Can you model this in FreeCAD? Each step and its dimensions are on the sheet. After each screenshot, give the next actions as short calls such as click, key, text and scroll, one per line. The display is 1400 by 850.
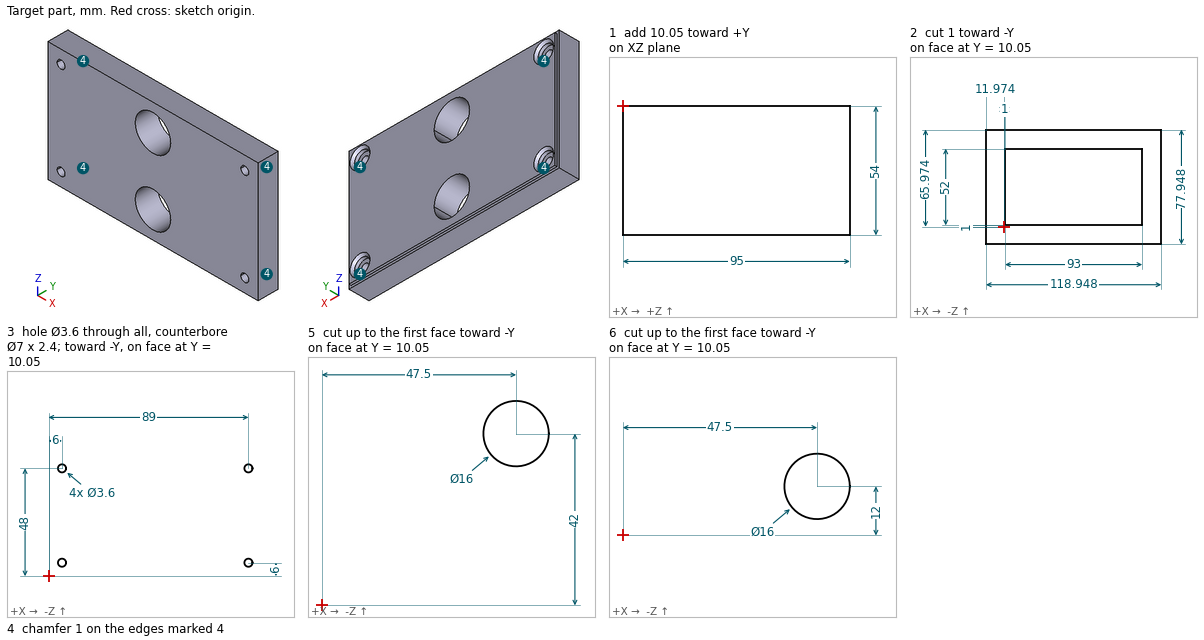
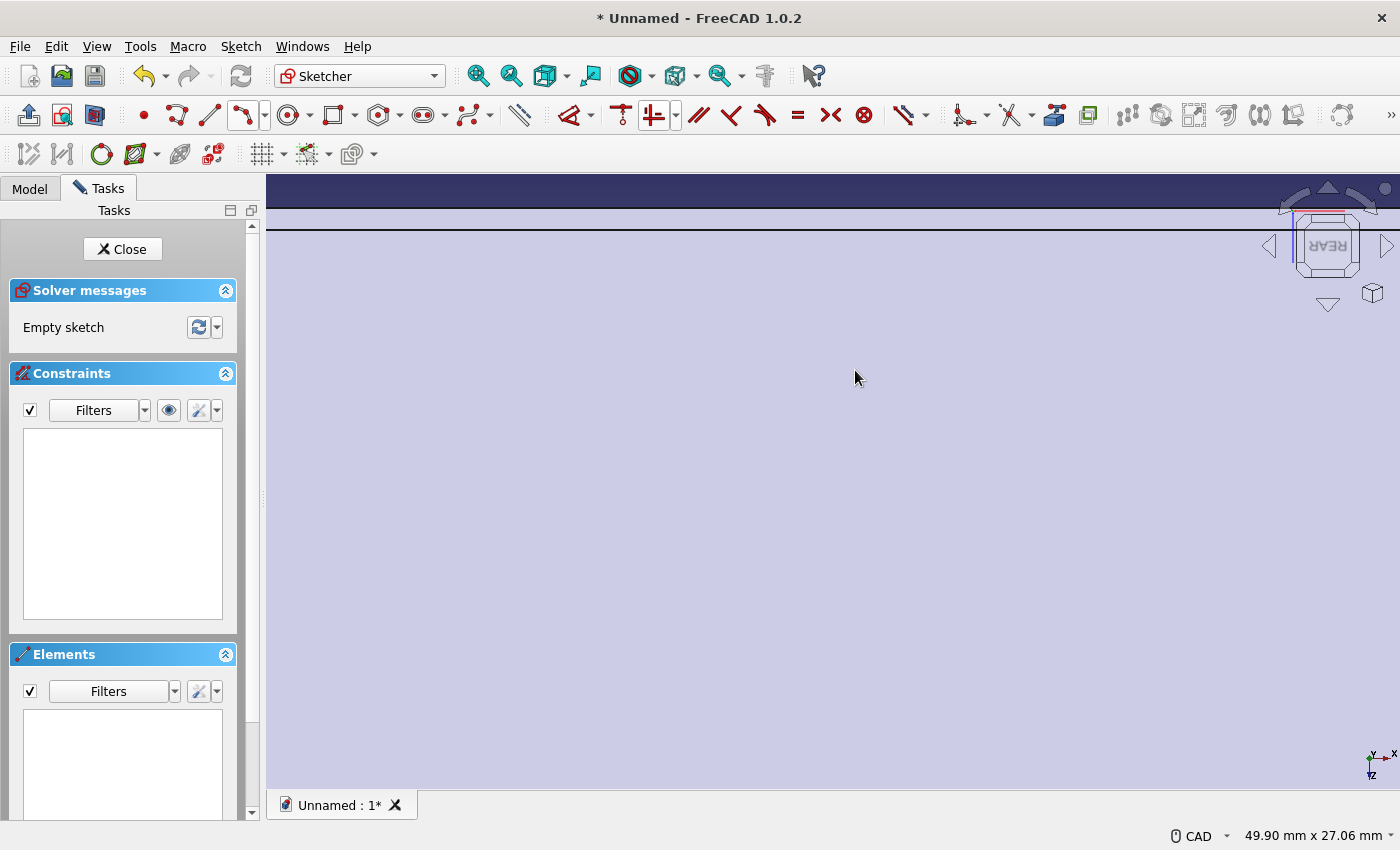
click(288, 116)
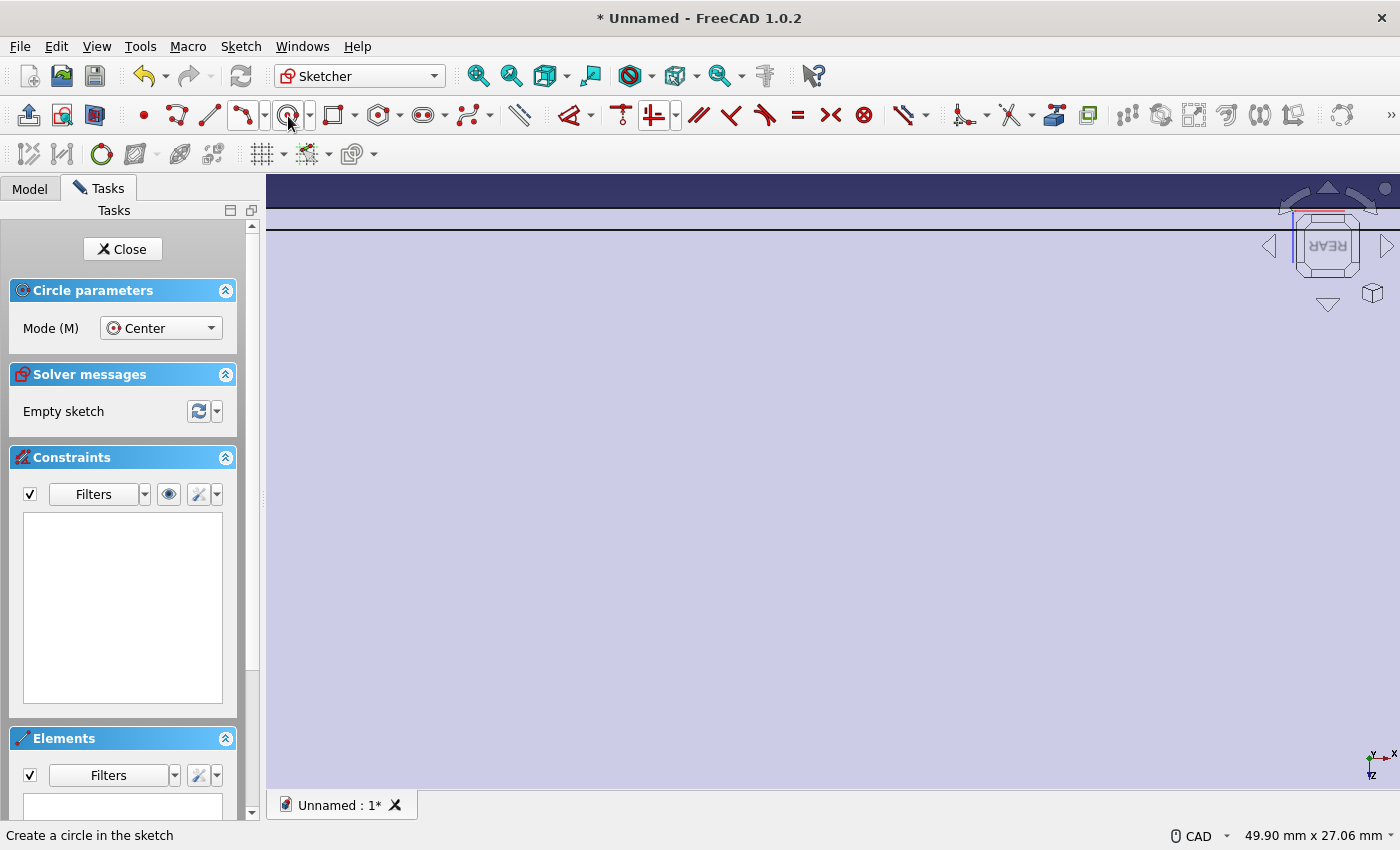
click(764, 480)
move(893, 352)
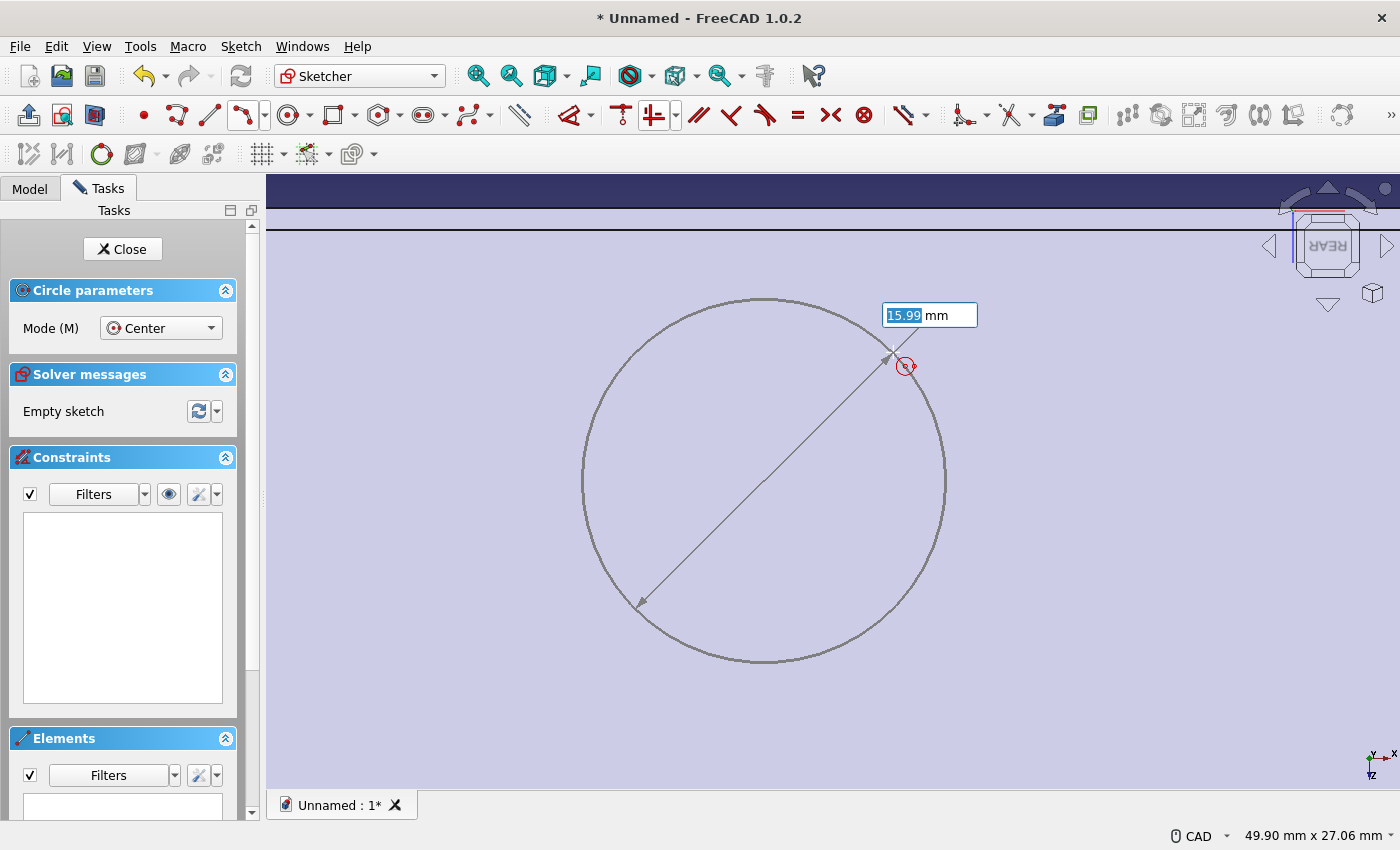
text(16)
key(Return)
key(Escape)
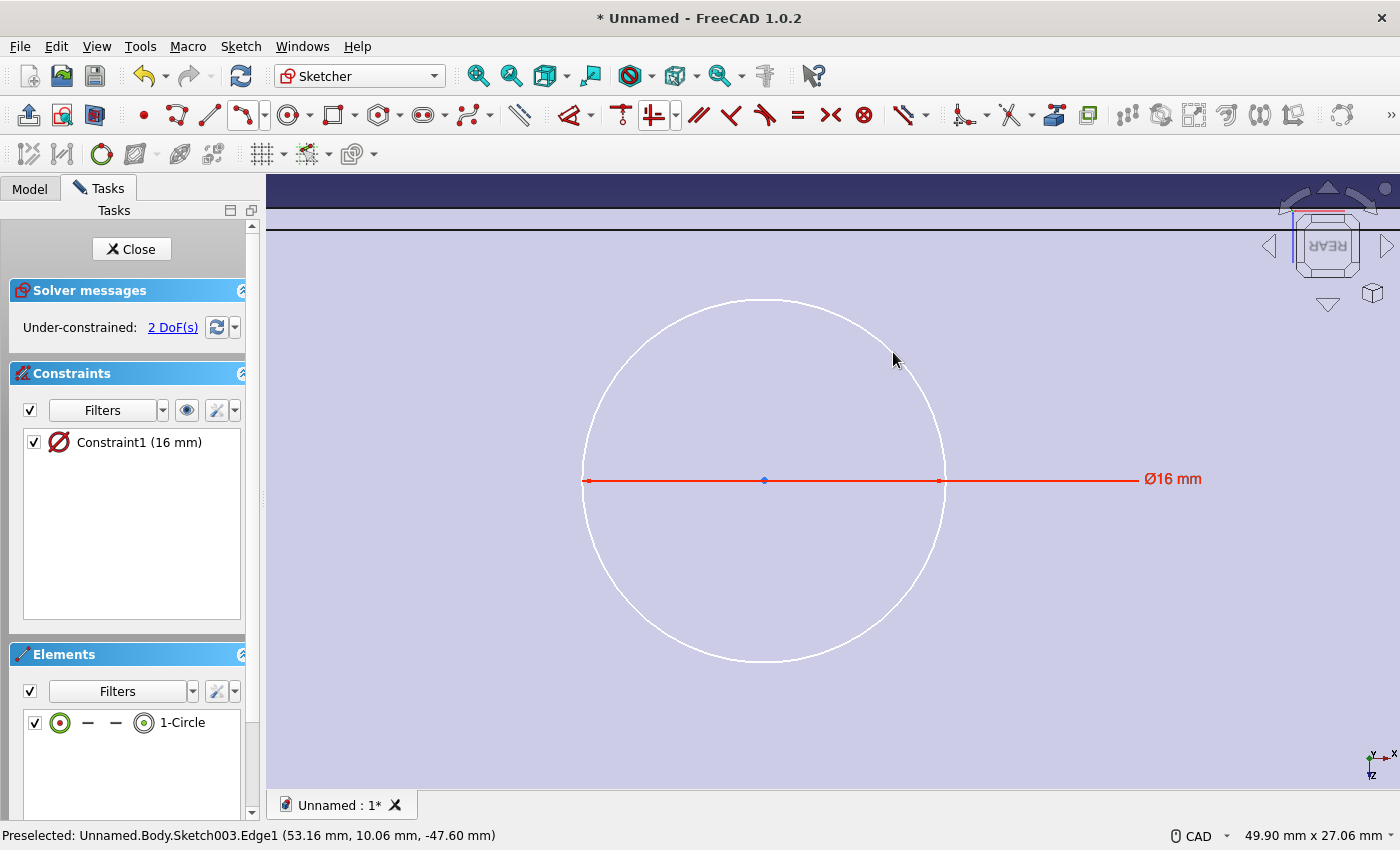
click(568, 116)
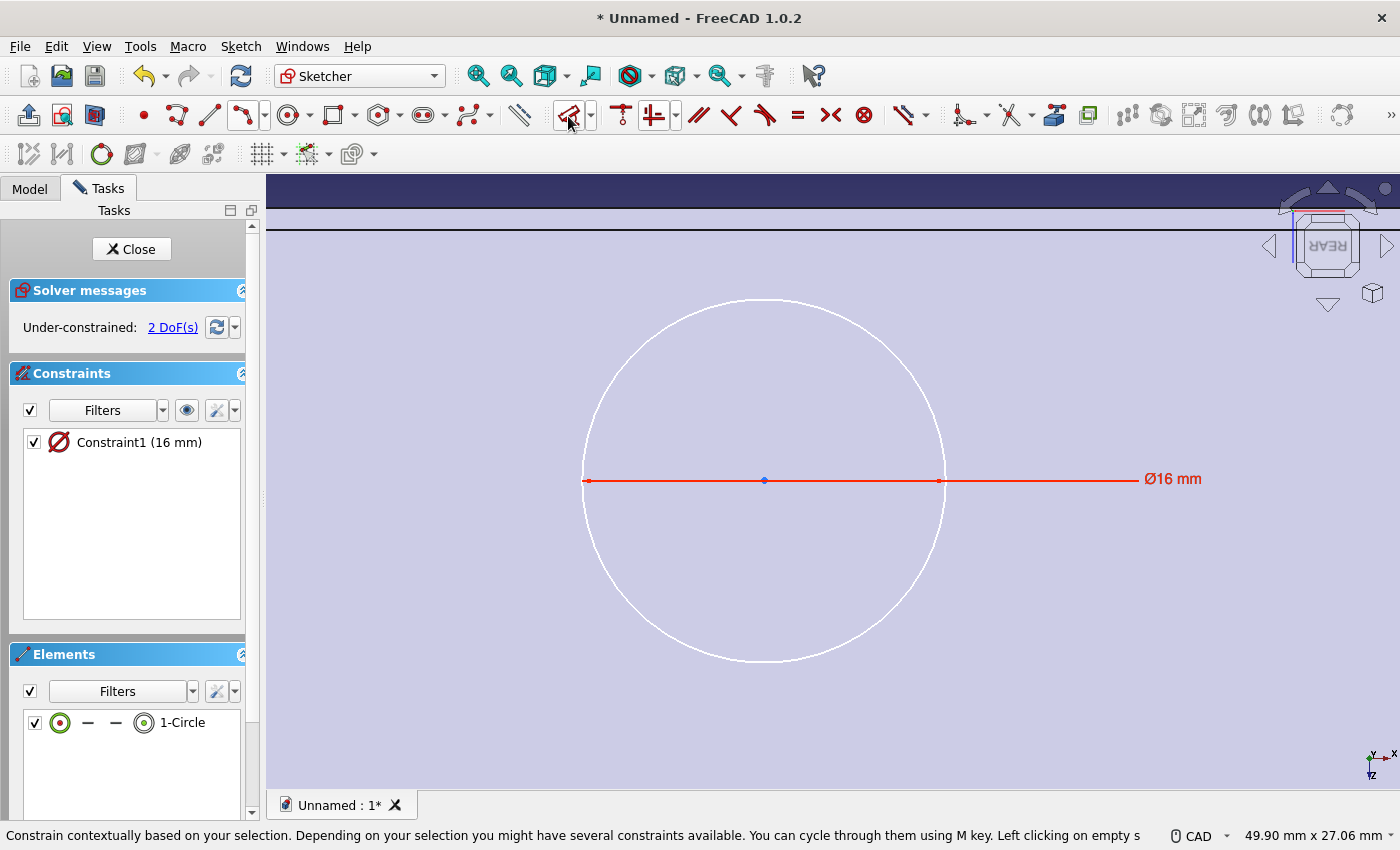
click(764, 481)
click(798, 621)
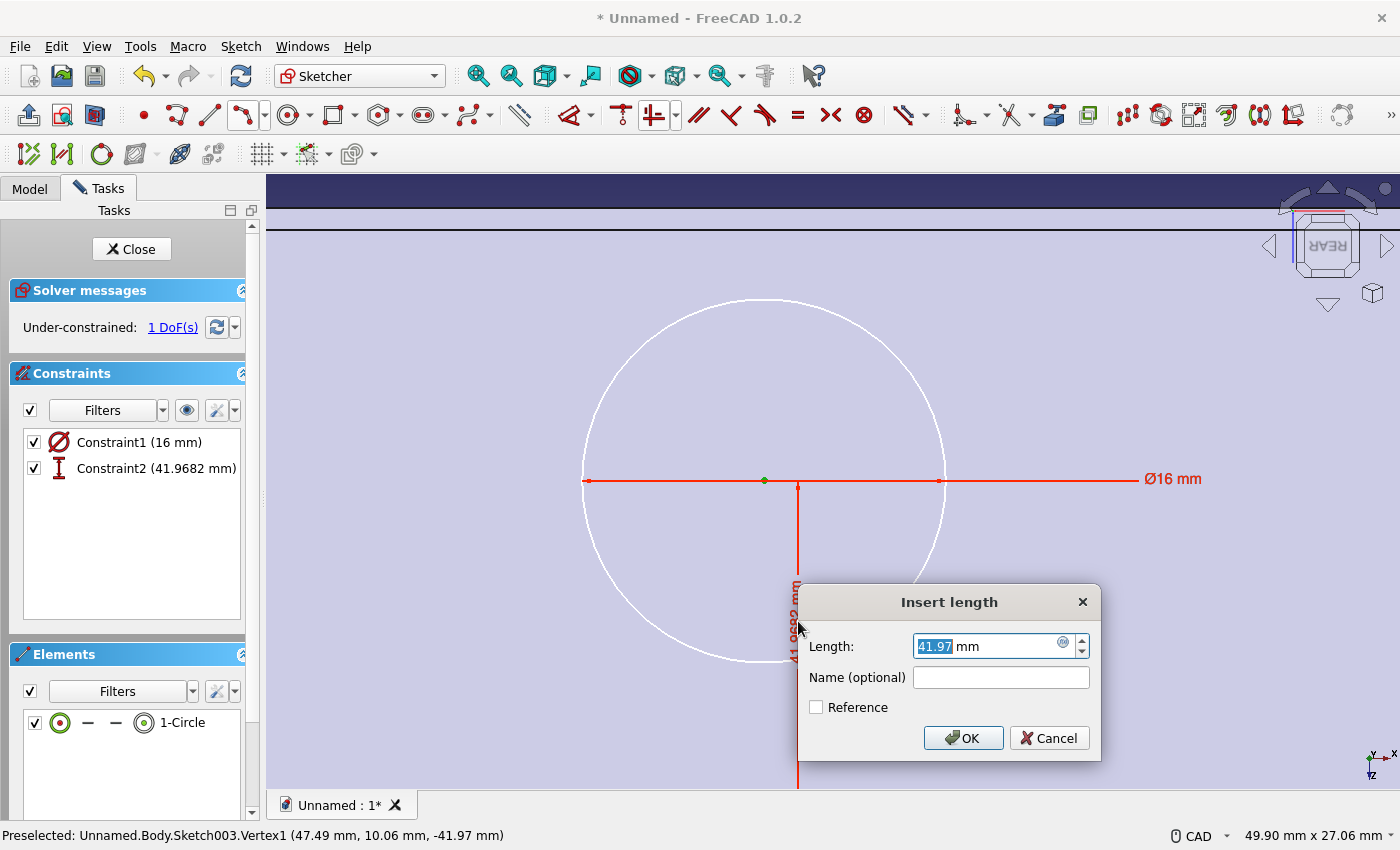
text(42)
key(Return)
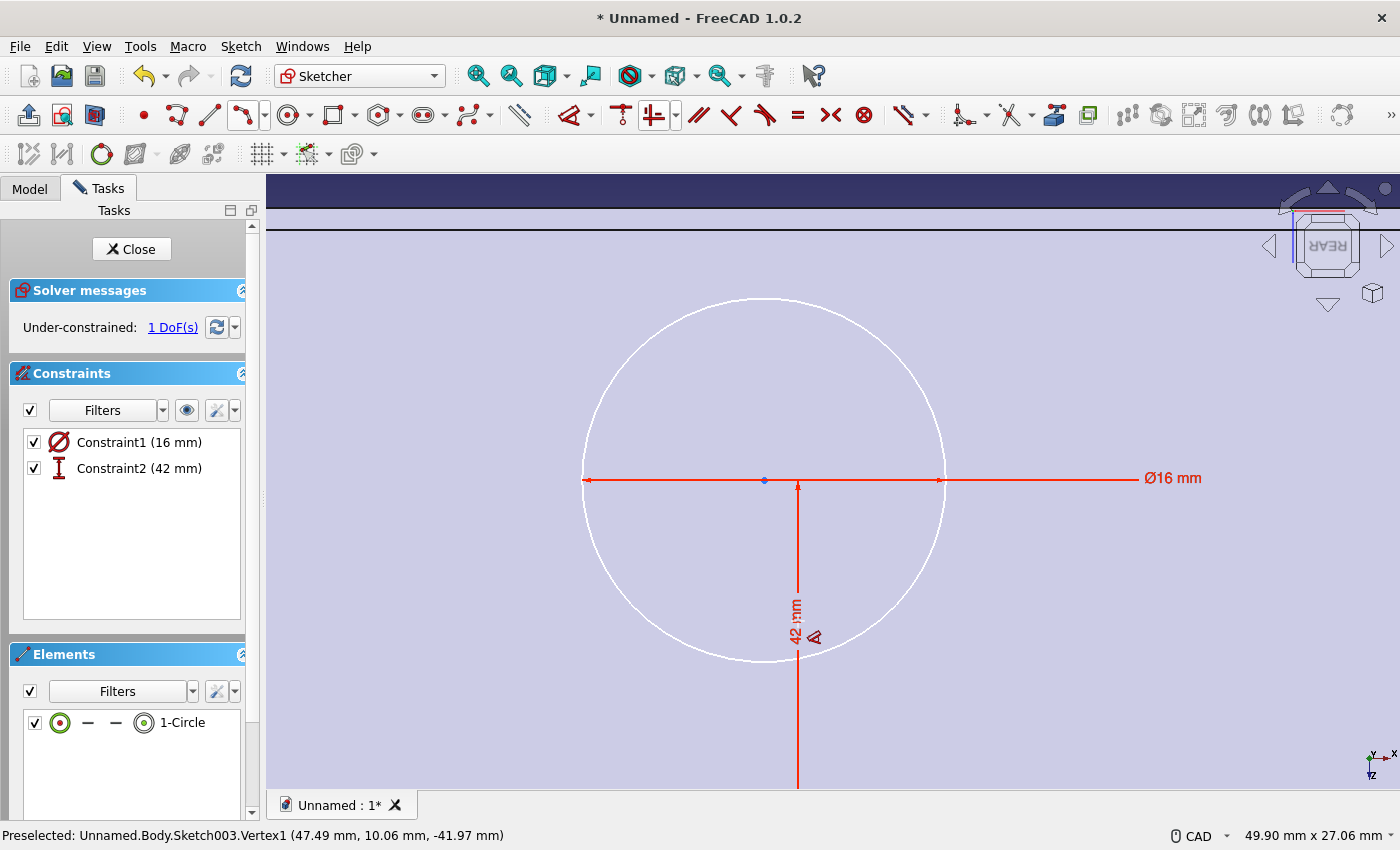
click(764, 480)
click(529, 446)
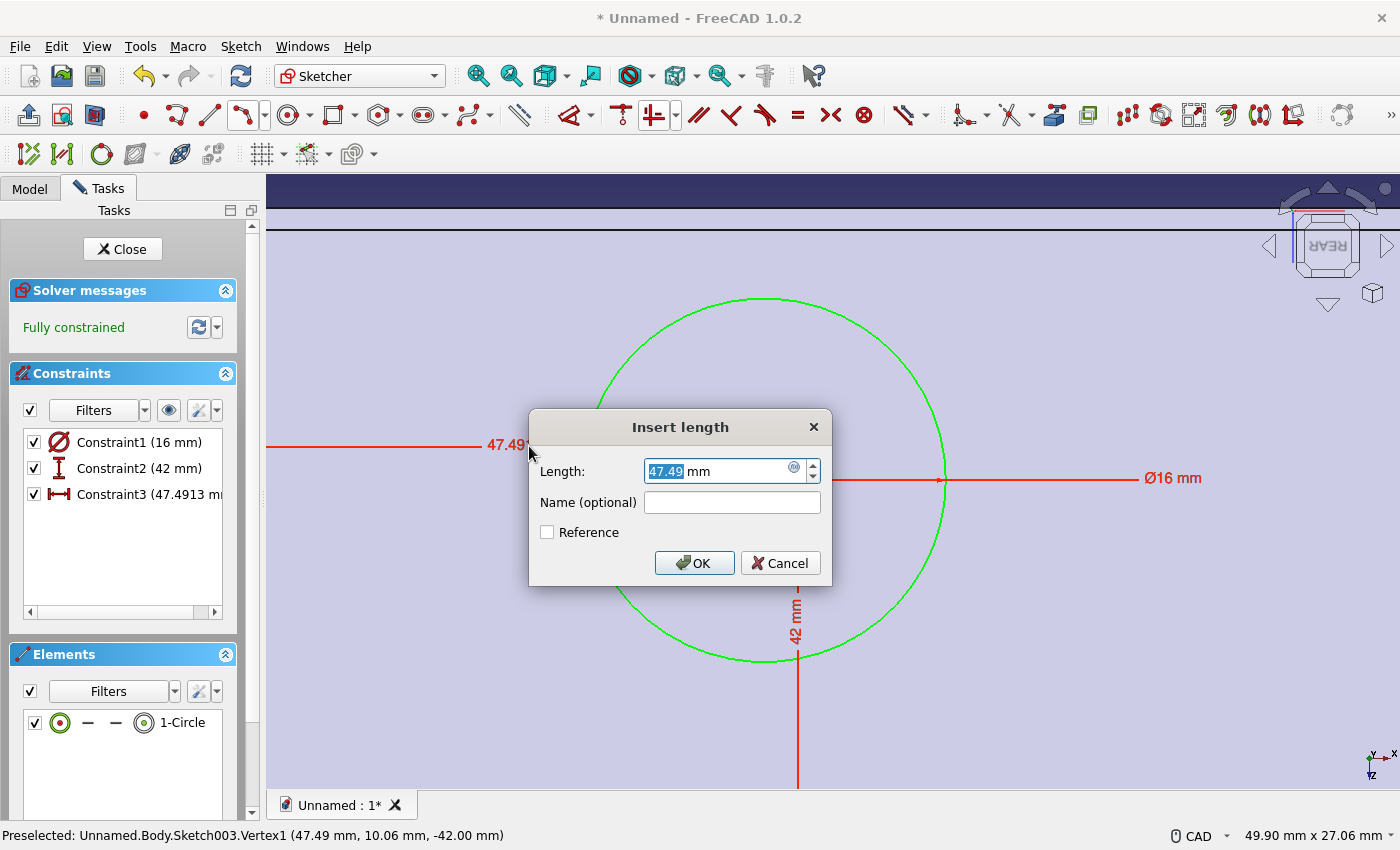
text(47.5)
key(Return)
key(Escape)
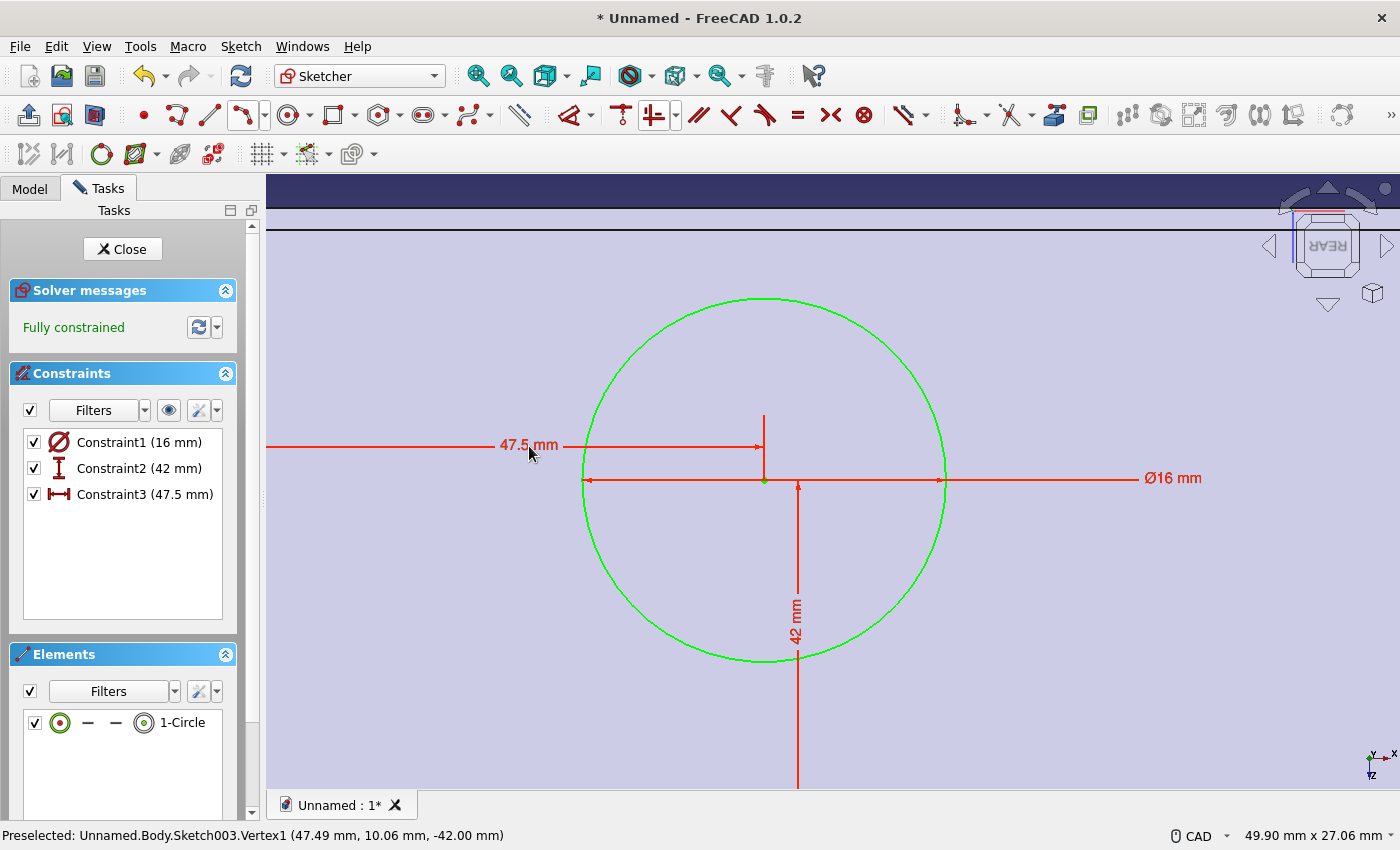
click(123, 249)